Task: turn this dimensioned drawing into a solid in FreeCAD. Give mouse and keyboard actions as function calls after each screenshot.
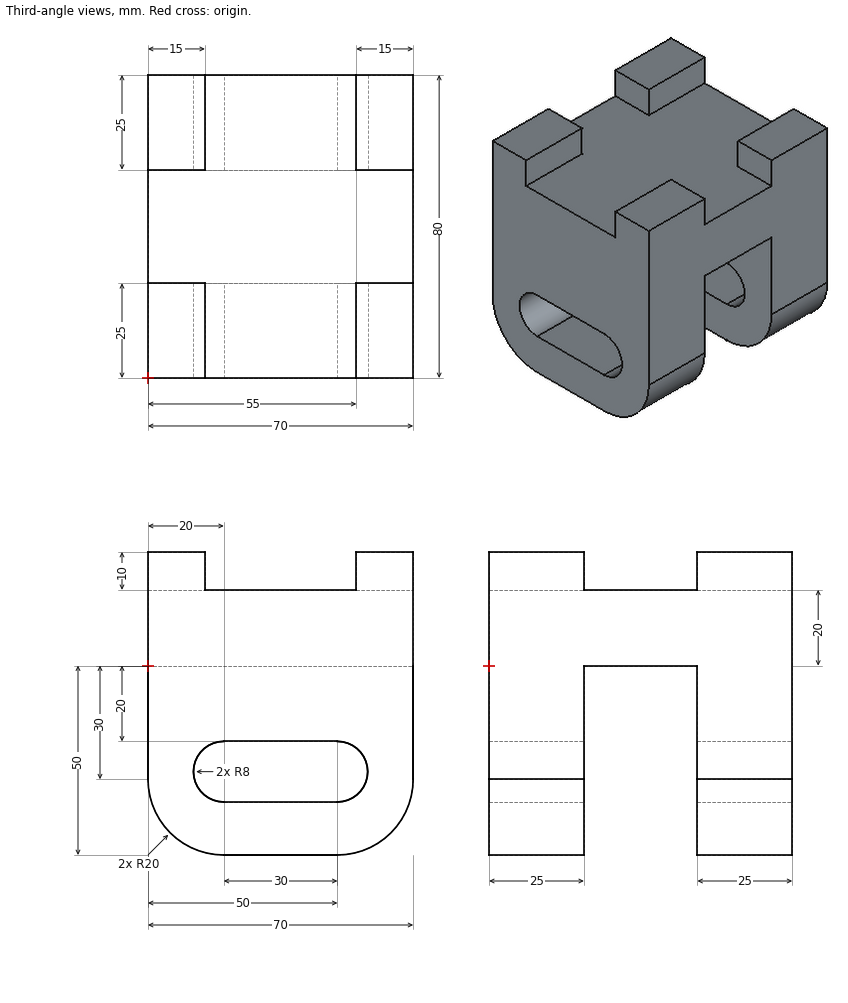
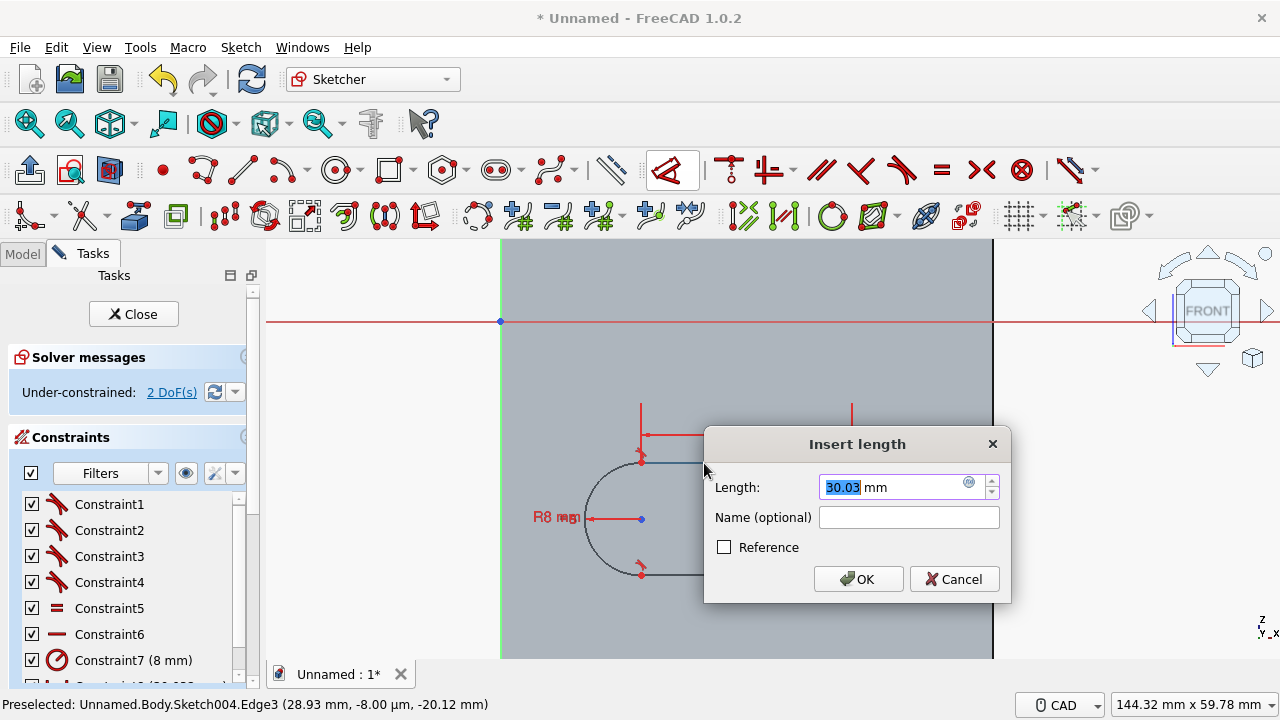
text(30)
key(Return)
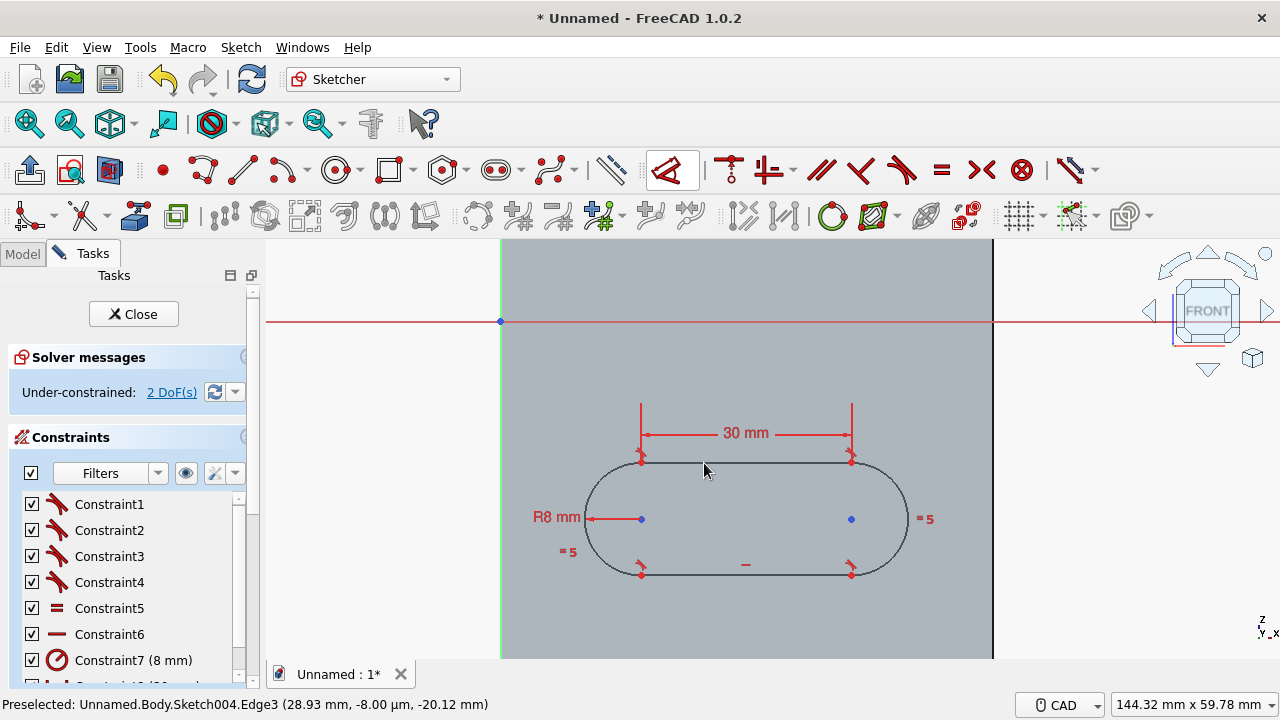
click(641, 463)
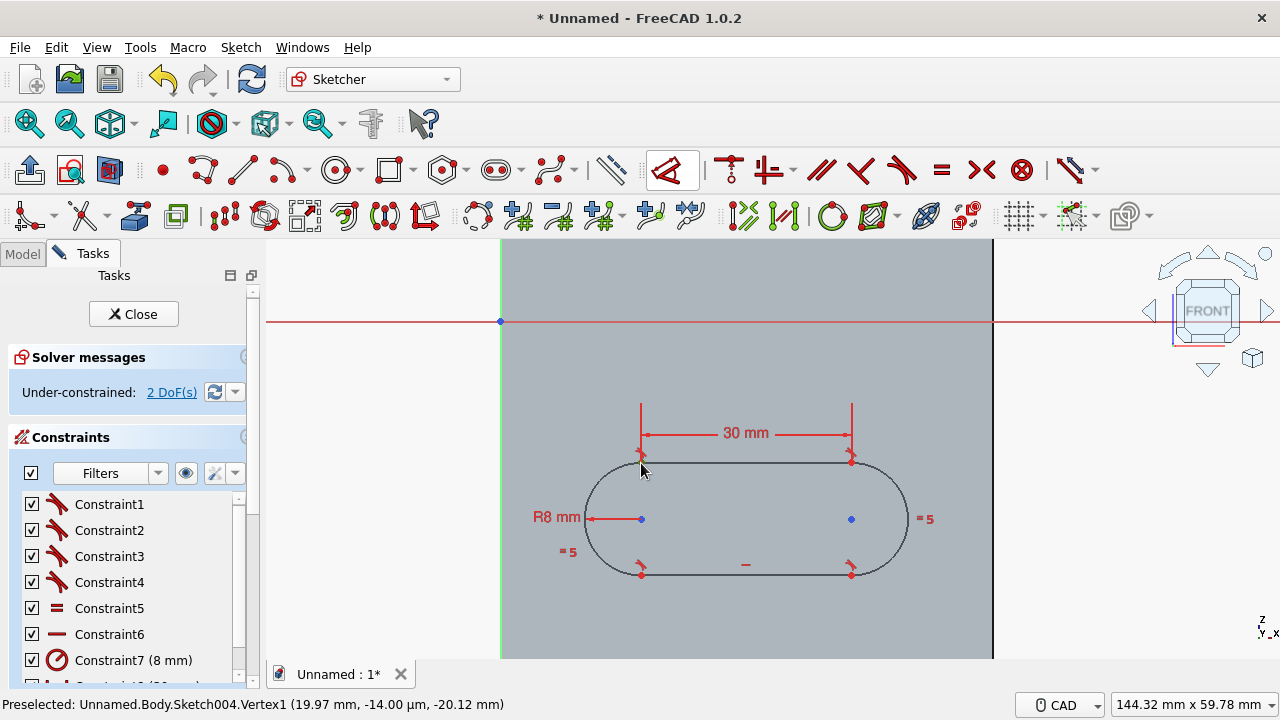
key(l)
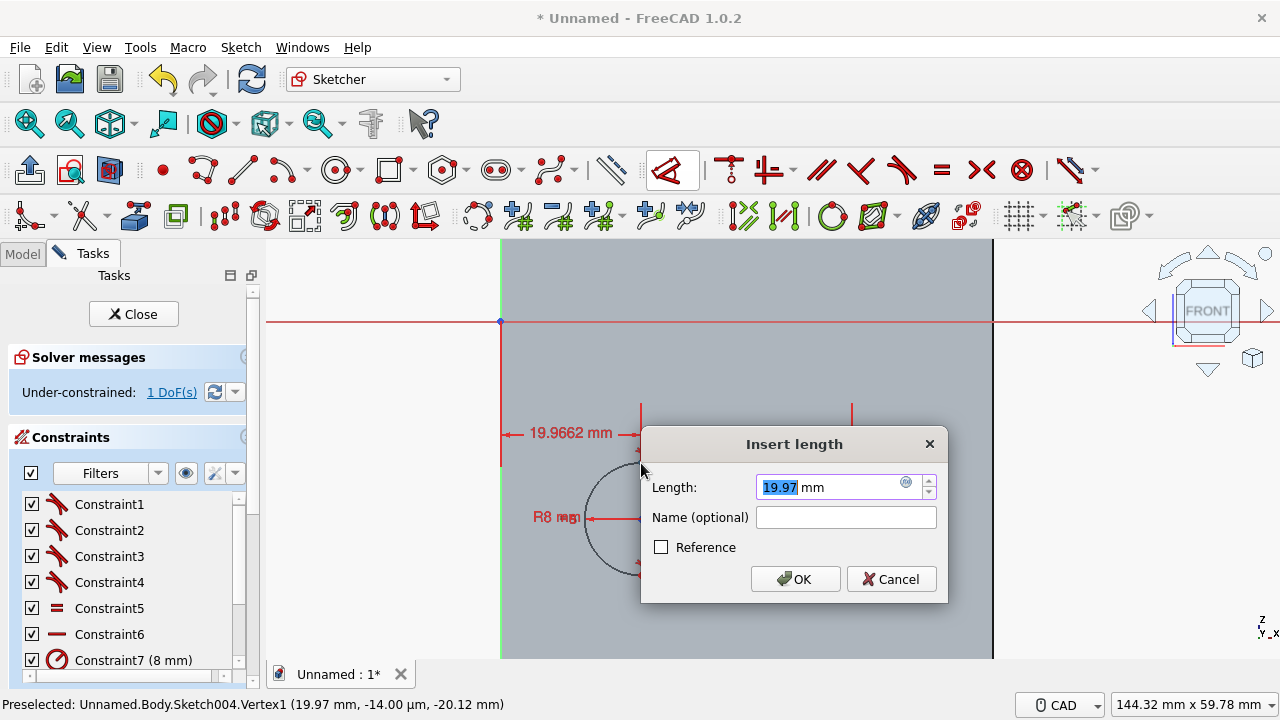
text(20)
key(Return)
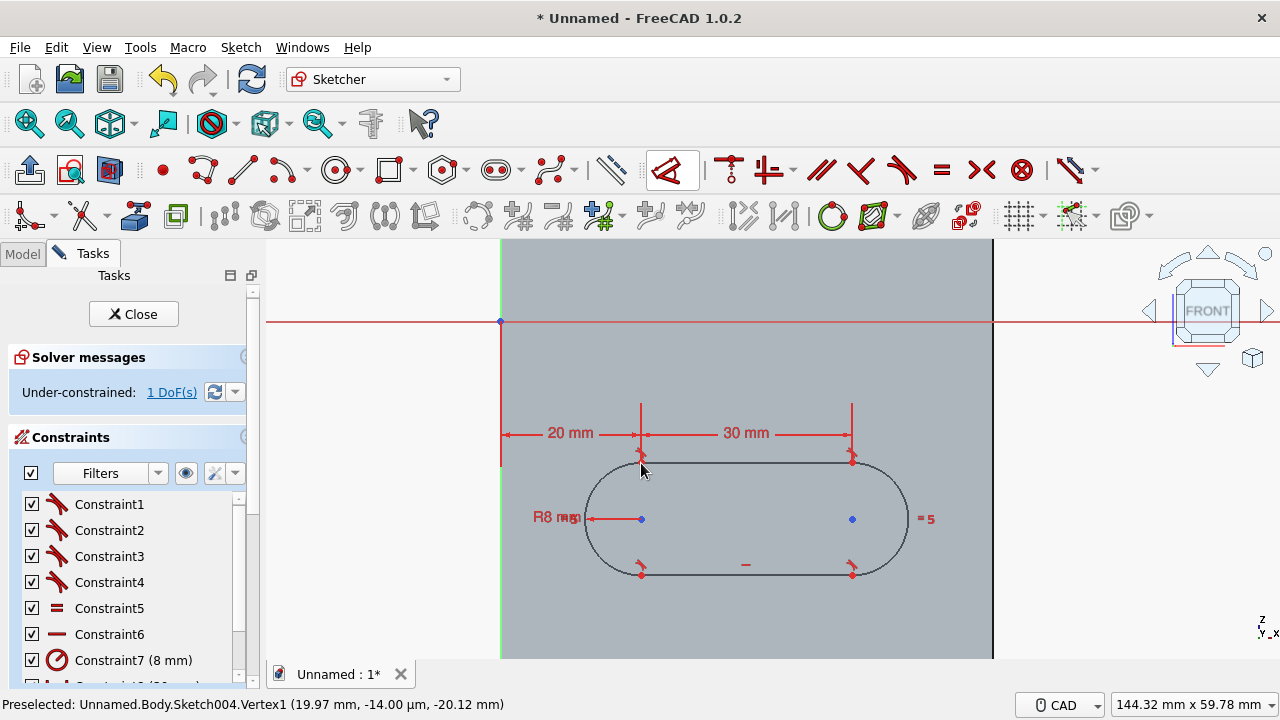
click(641, 463)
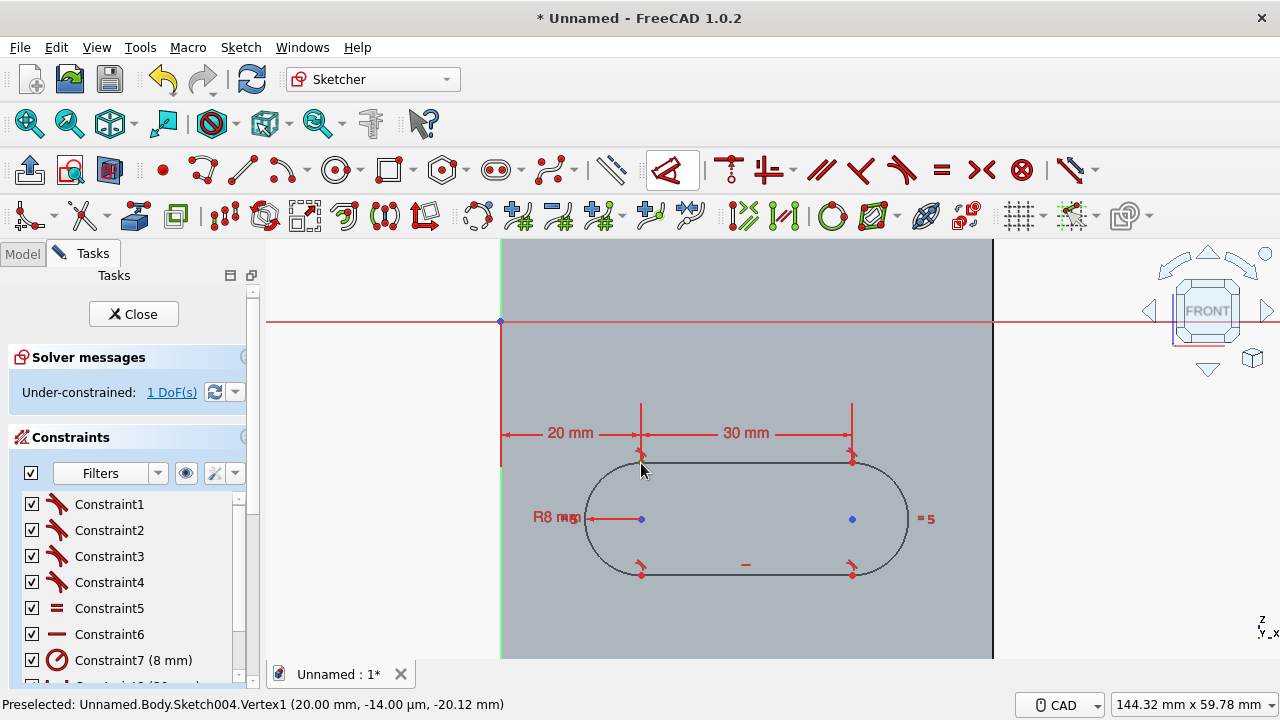
key(i)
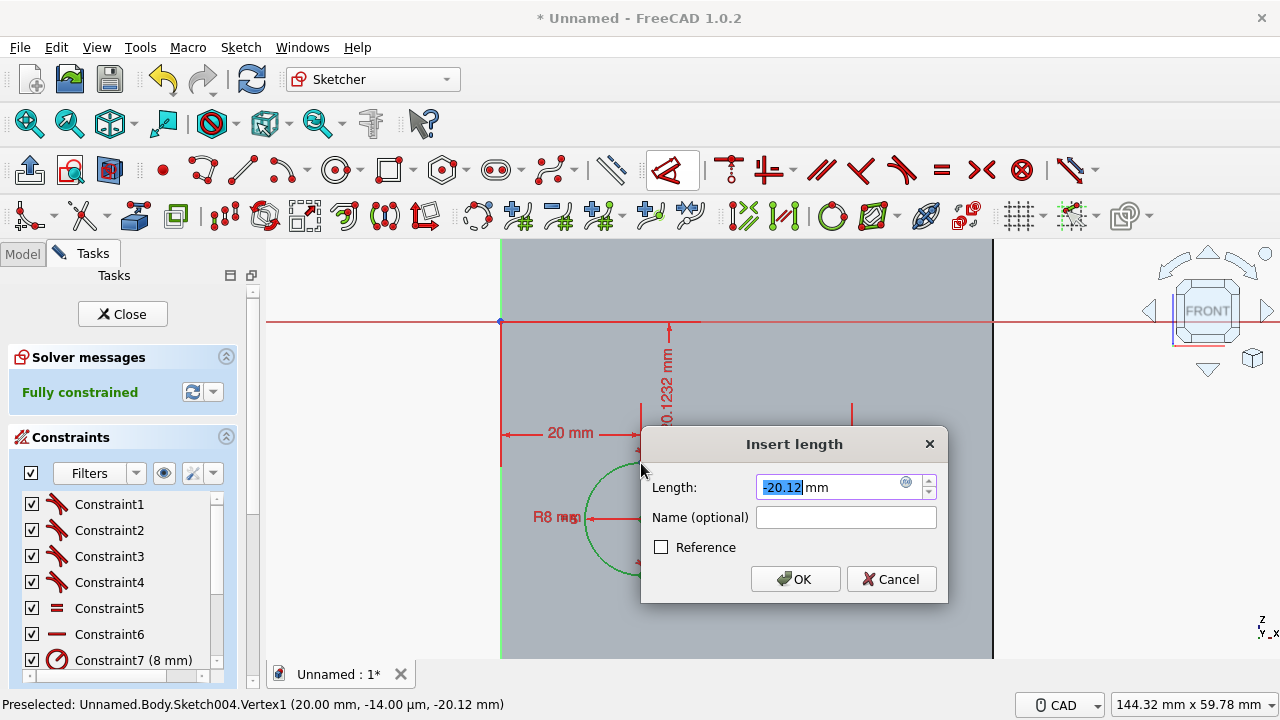
text(-20)
key(Return)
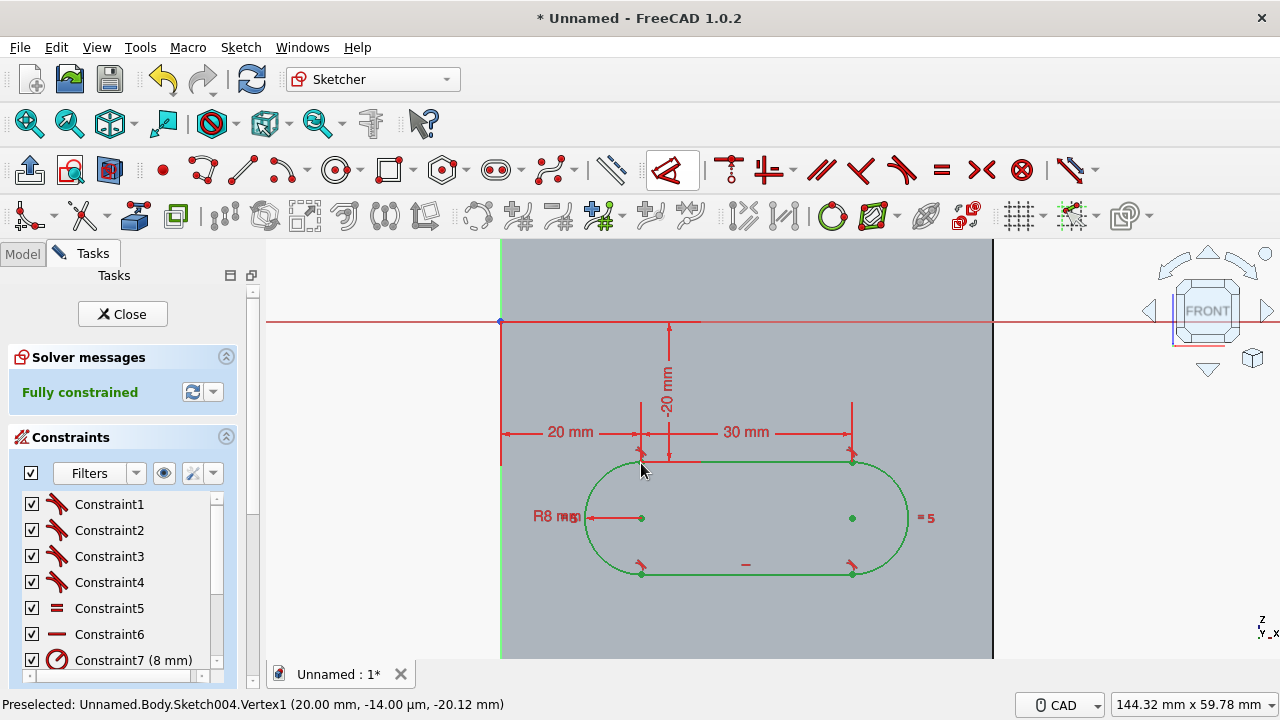
click(123, 314)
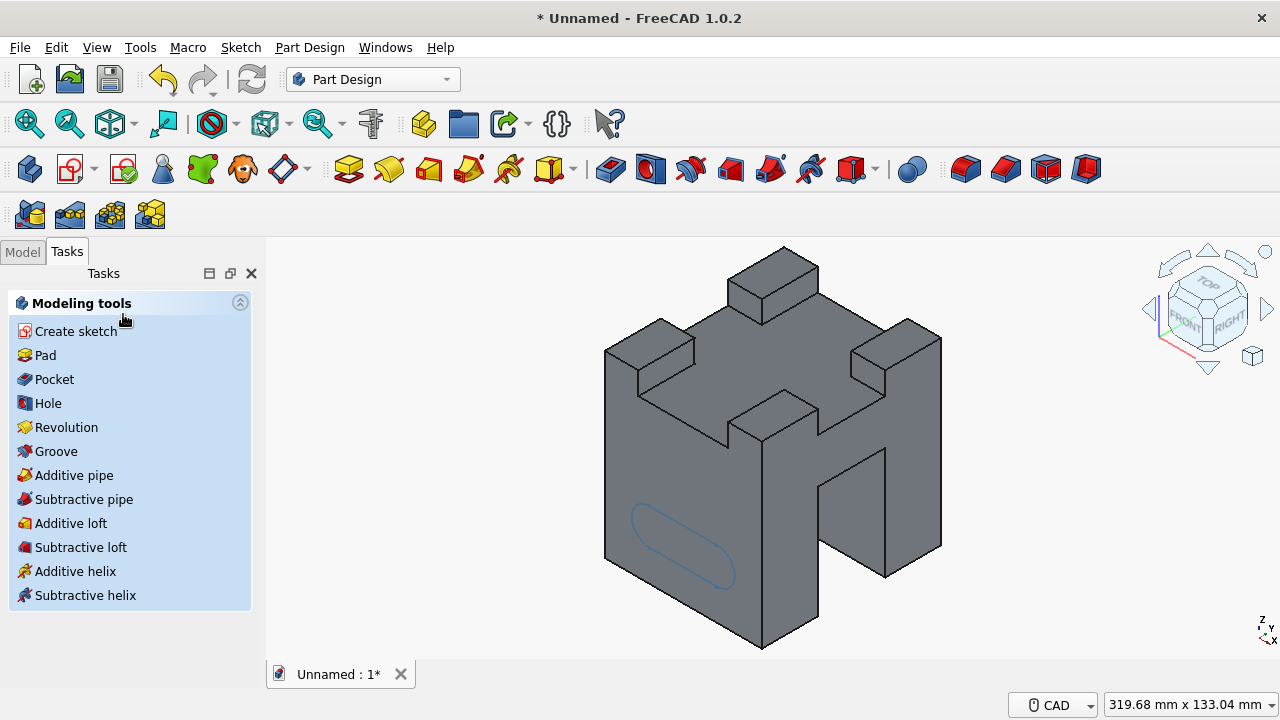
click(612, 170)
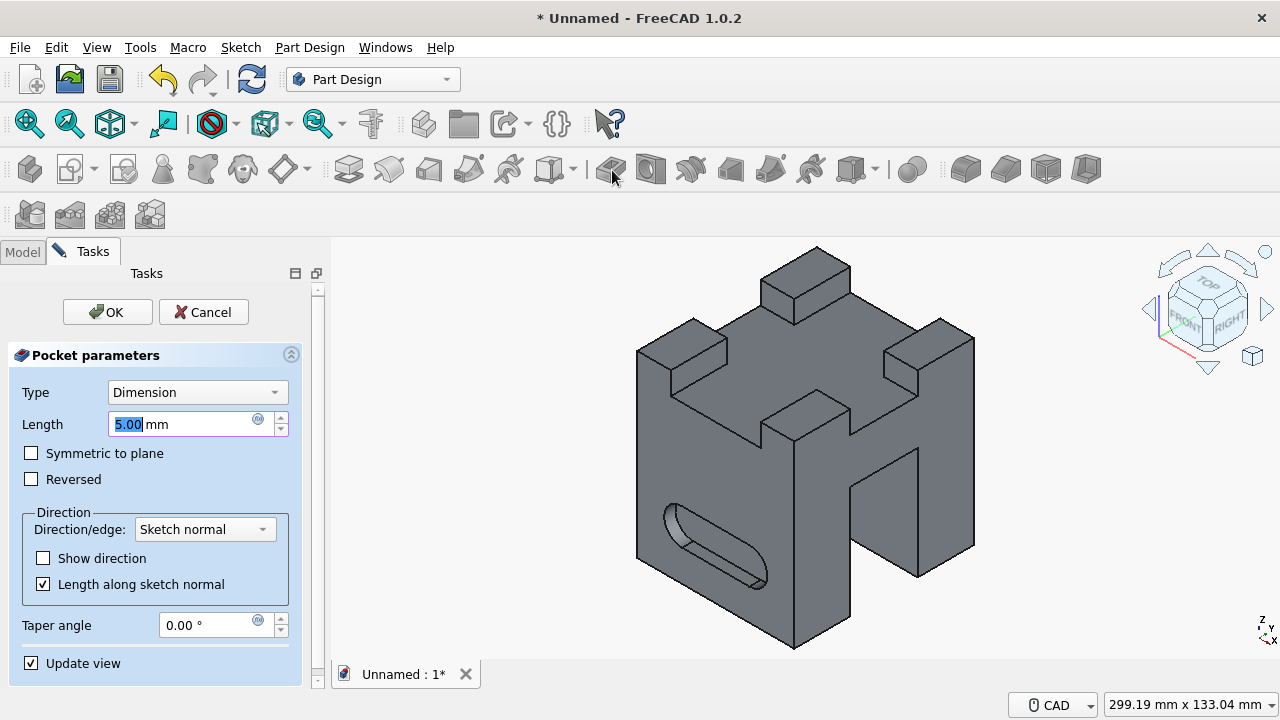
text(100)
key(Tab)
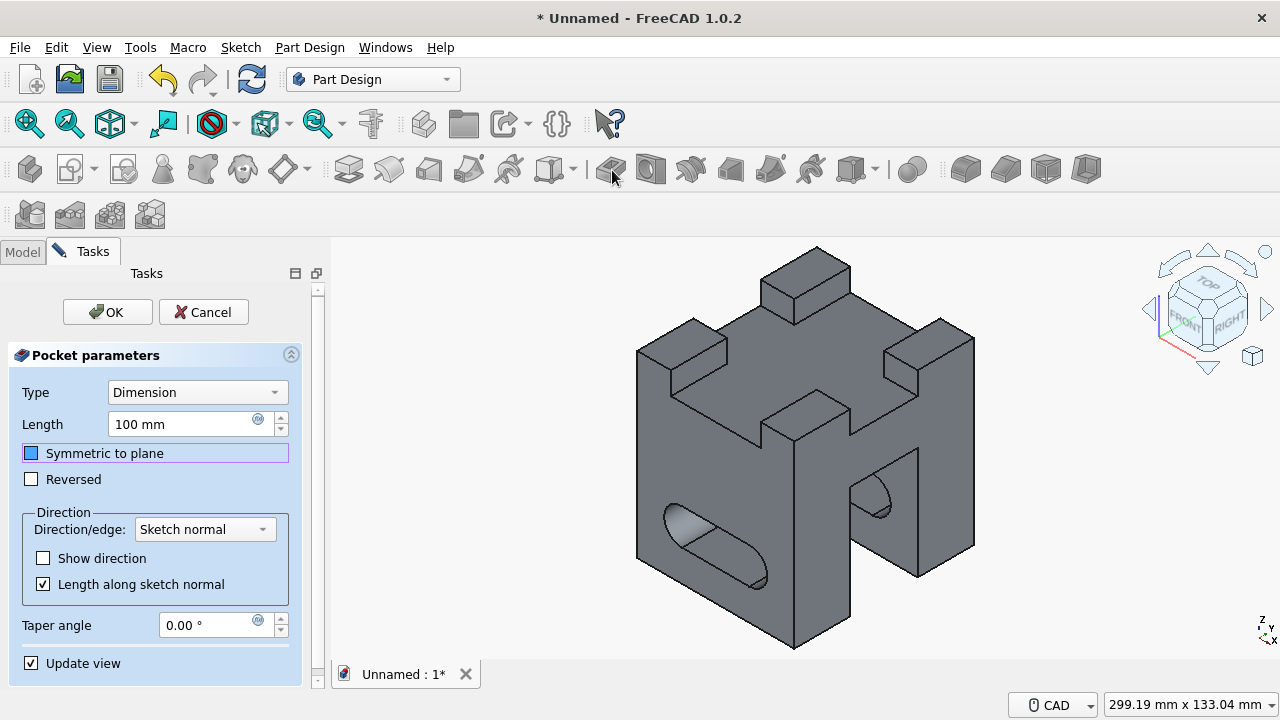
click(108, 312)